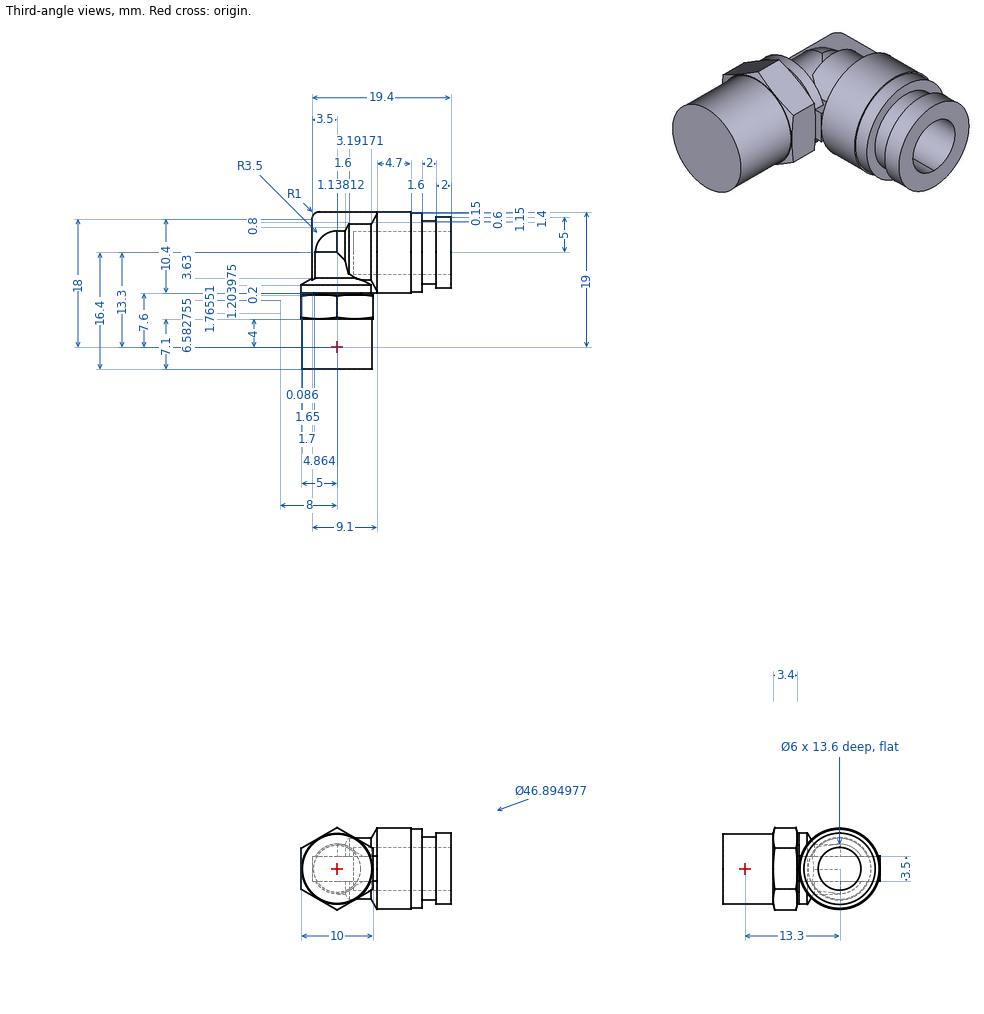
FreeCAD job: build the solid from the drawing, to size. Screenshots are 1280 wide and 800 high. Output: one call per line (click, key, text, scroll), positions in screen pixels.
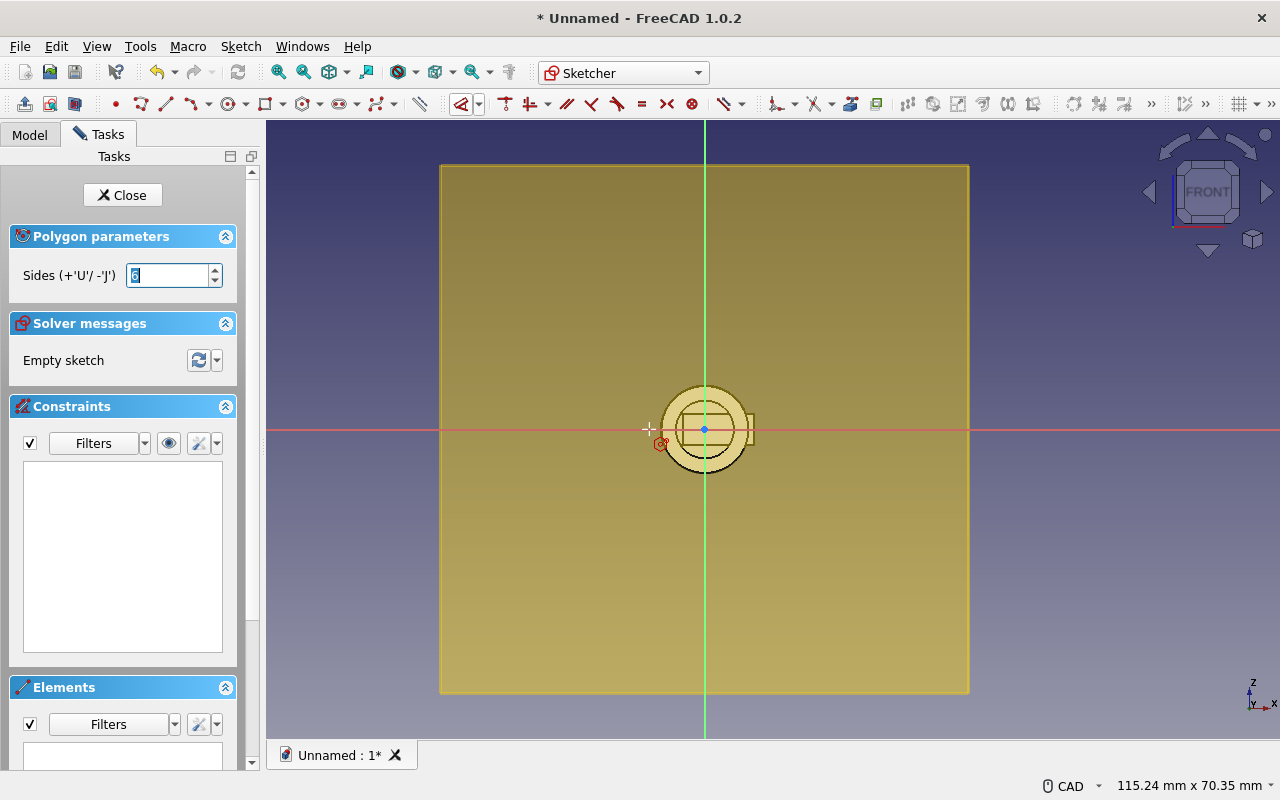
click(705, 430)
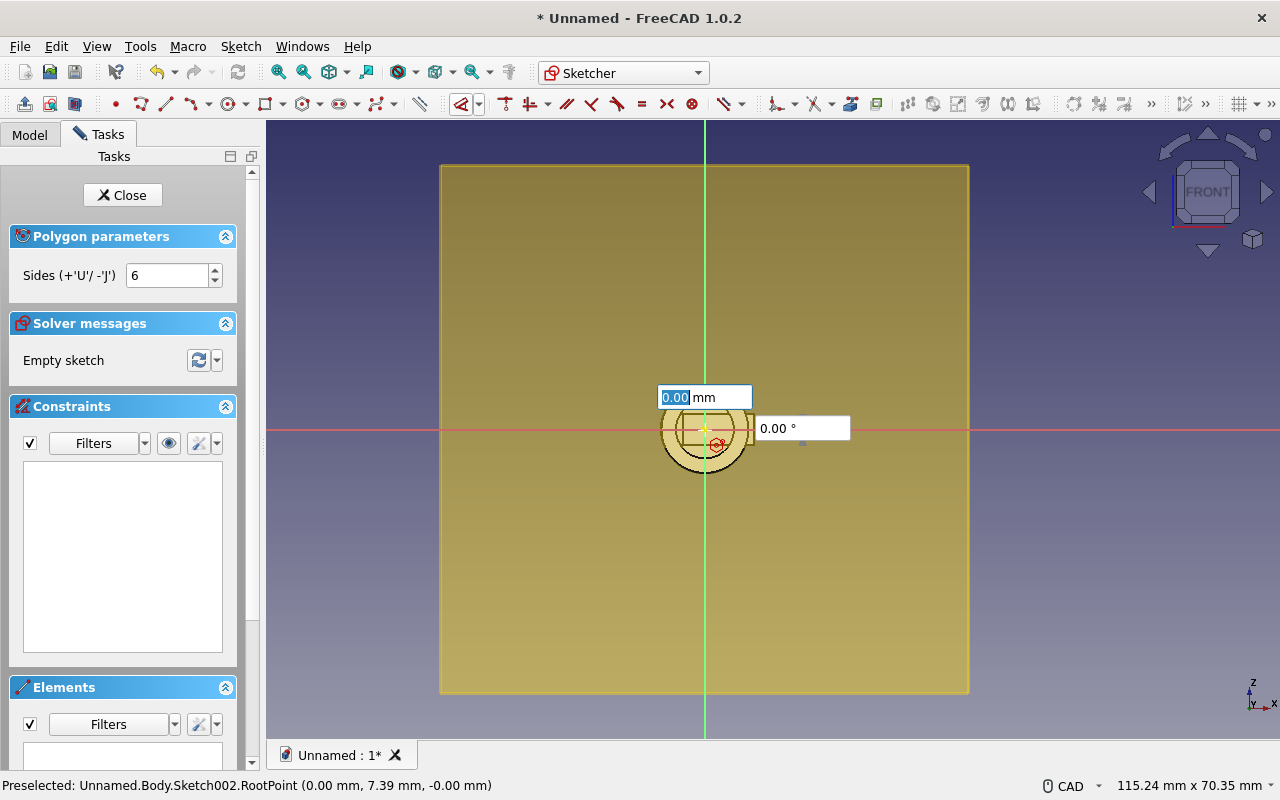
click(705, 480)
key(Escape)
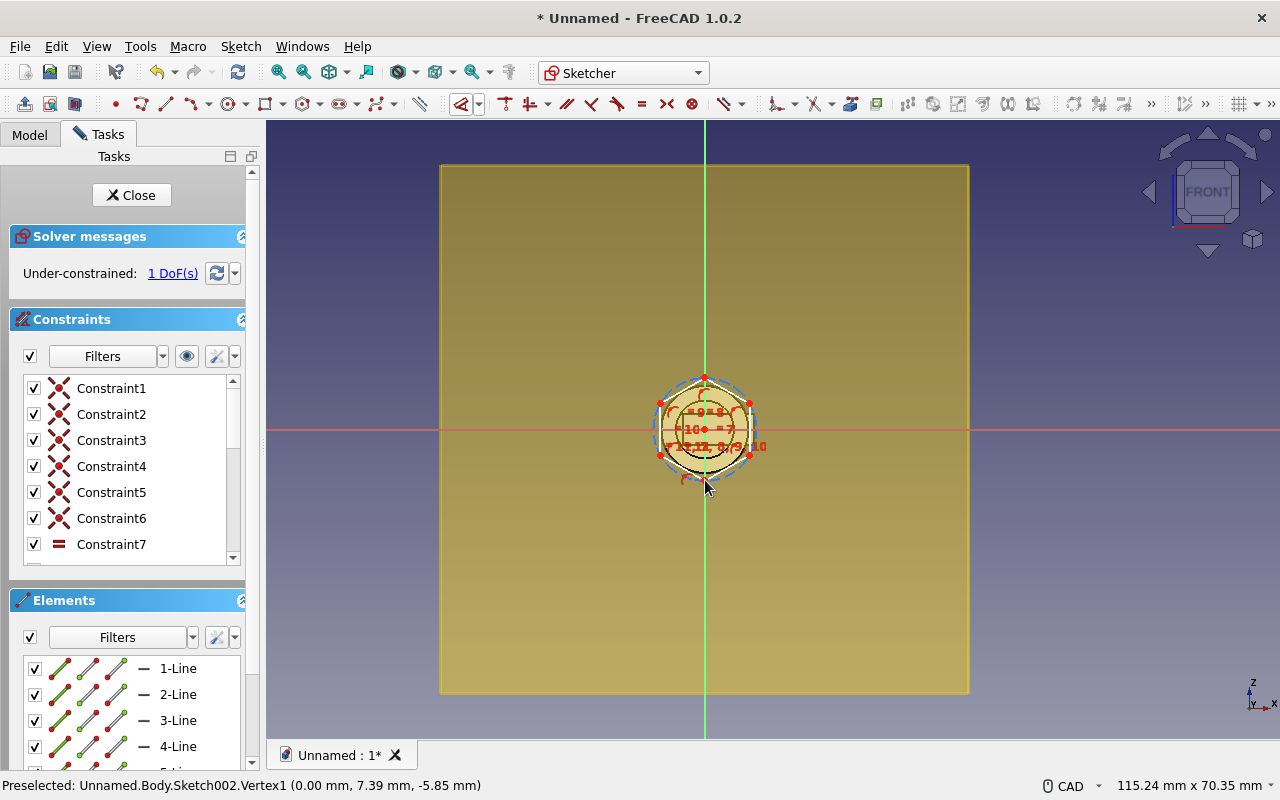
click(228, 104)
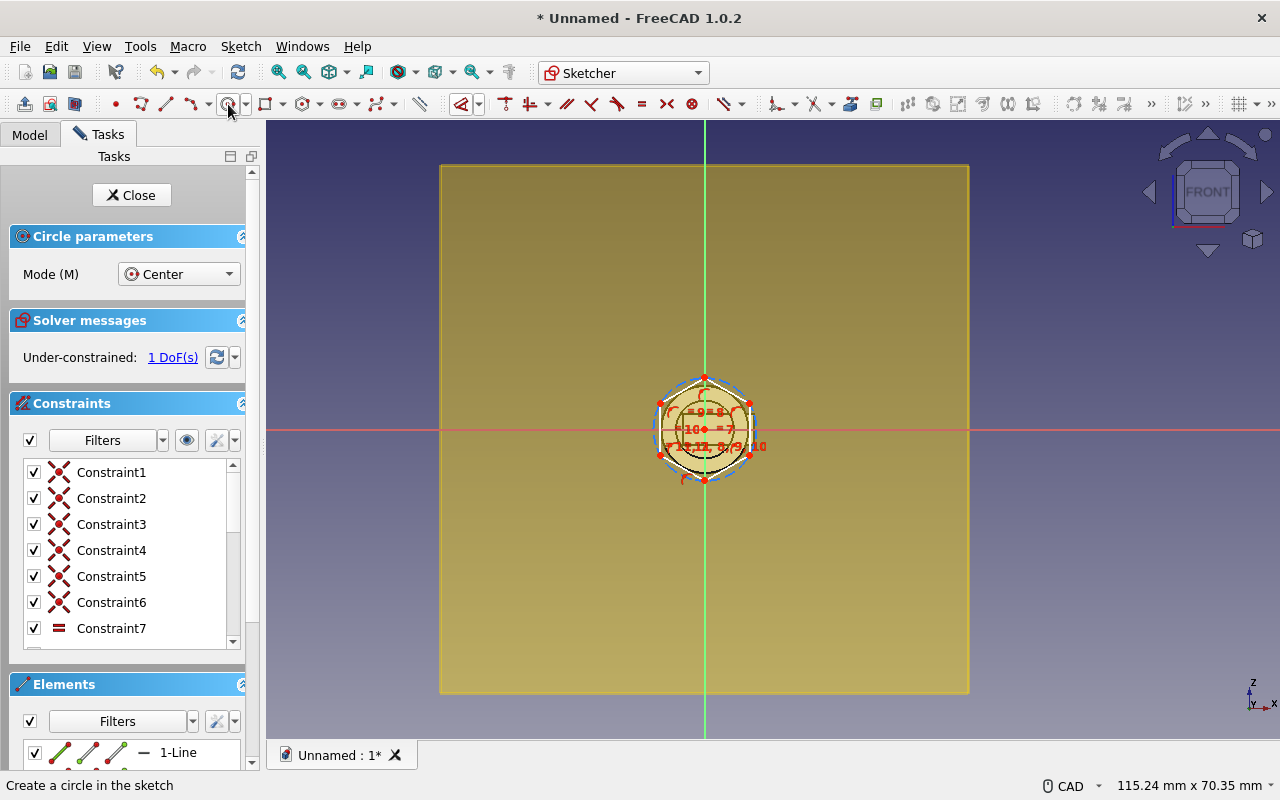
click(705, 430)
click(851, 284)
key(Escape)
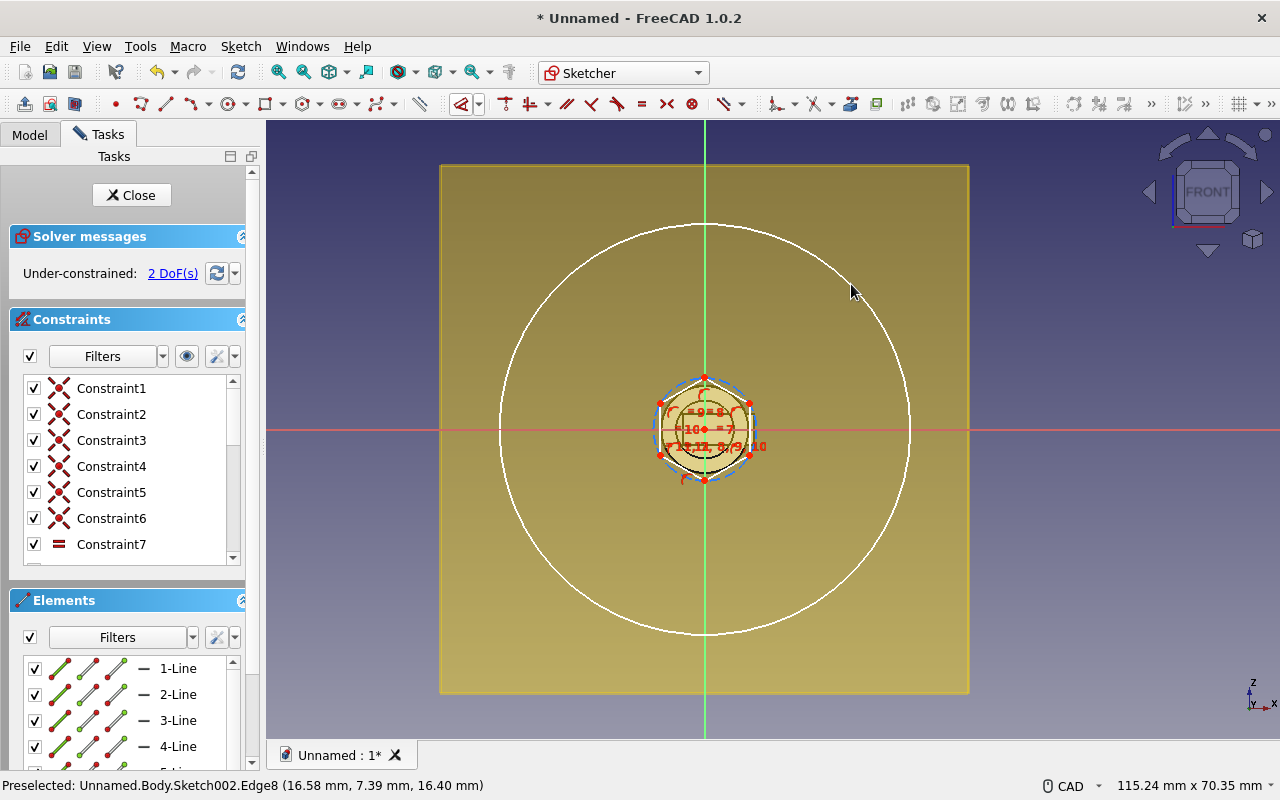
click(850, 284)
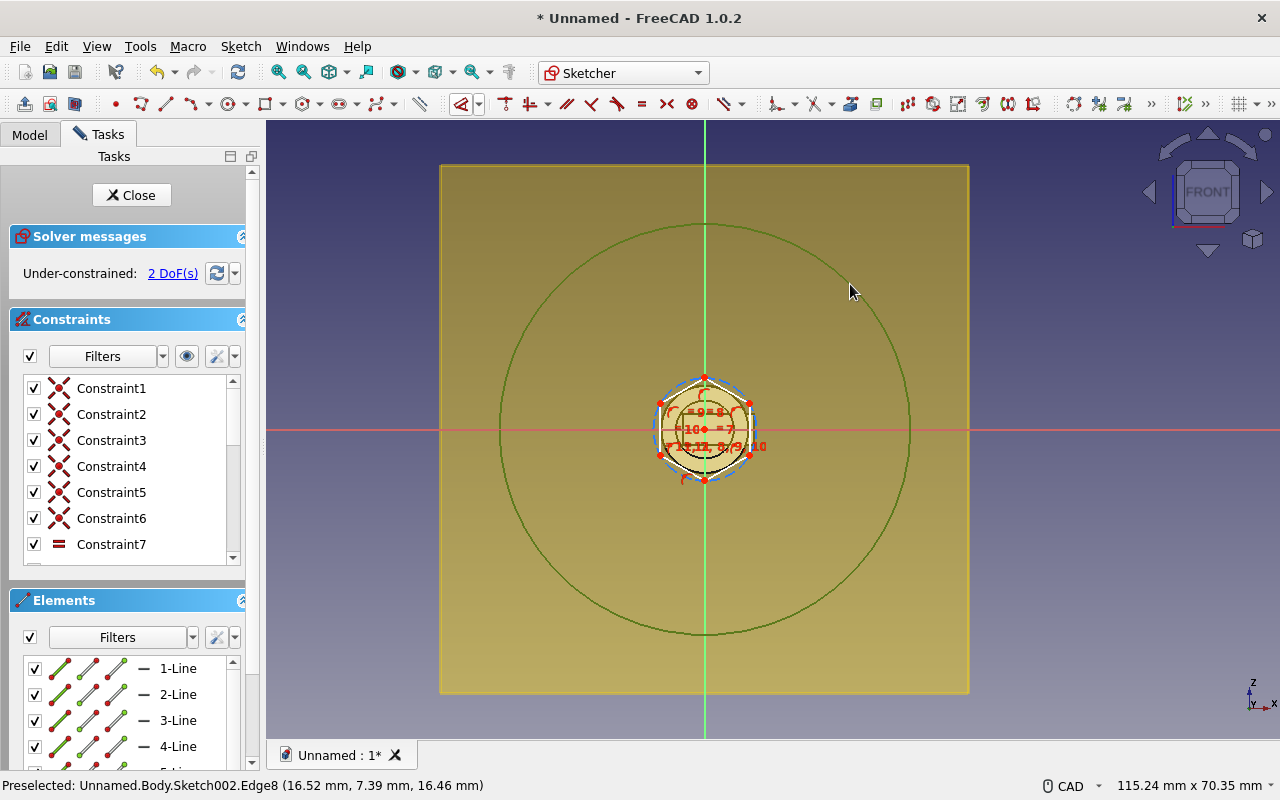
key(k)
key(o)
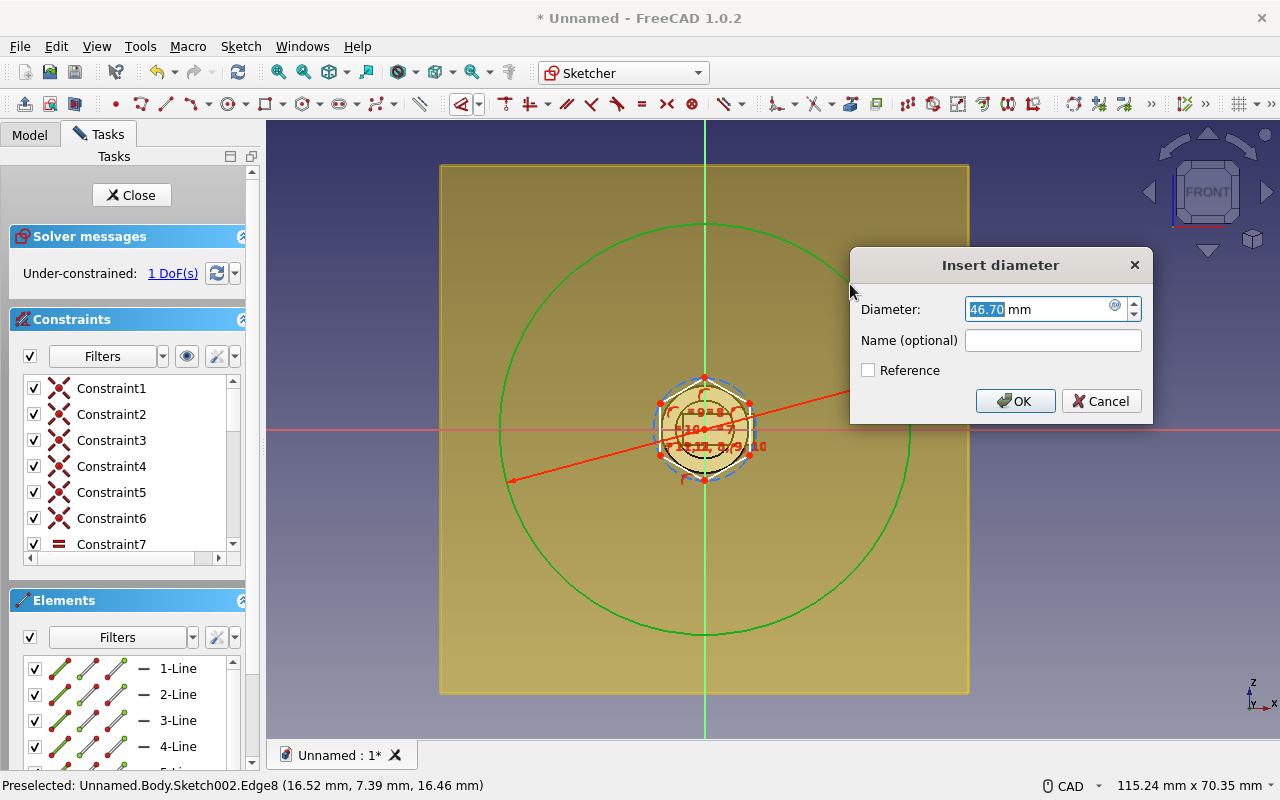
text(46.894977)
key(Return)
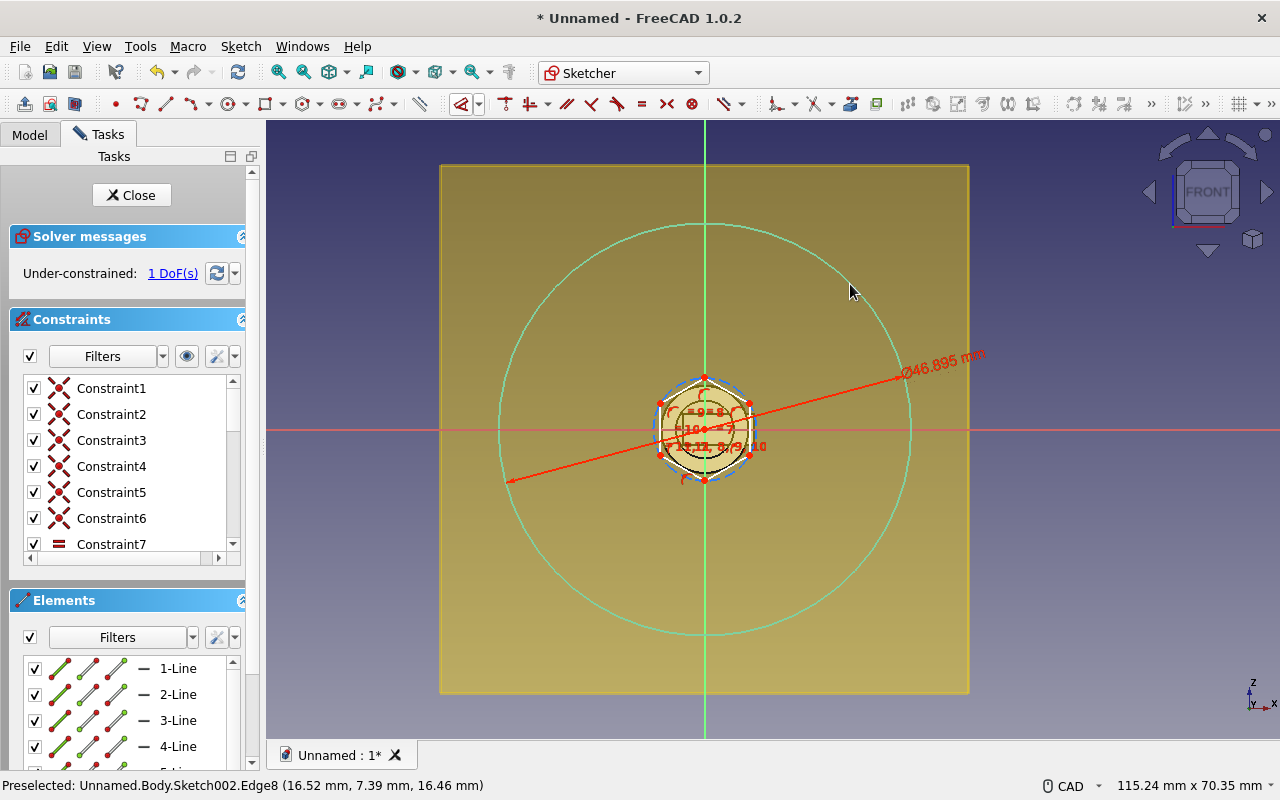
click(660, 404)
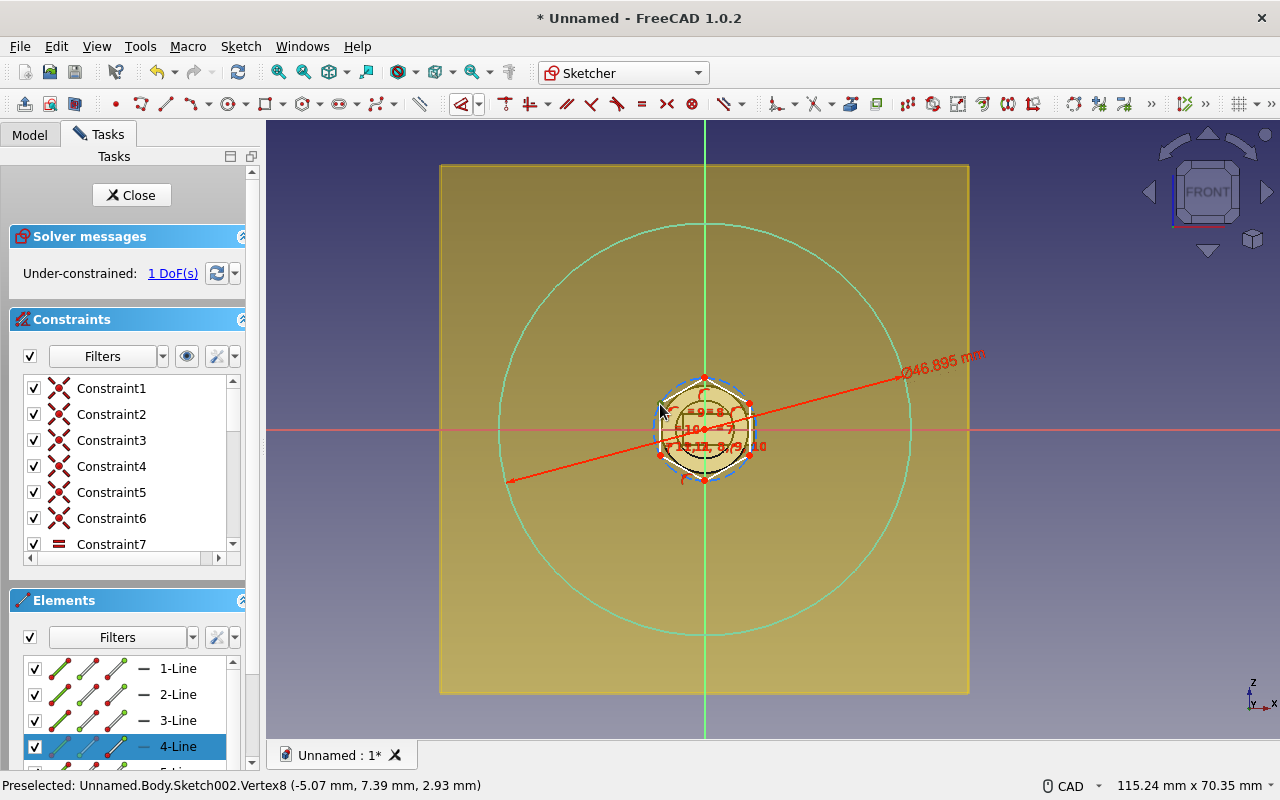
click(750, 455)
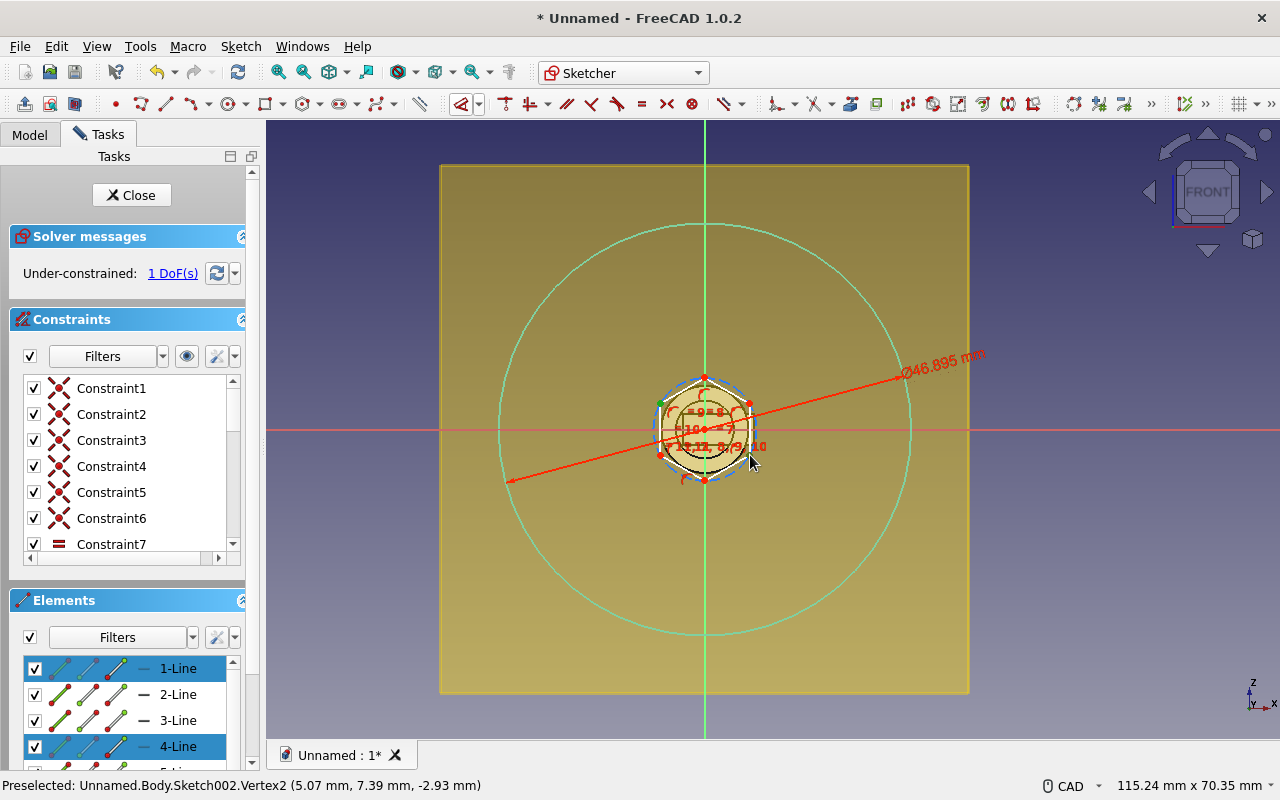
click(478, 104)